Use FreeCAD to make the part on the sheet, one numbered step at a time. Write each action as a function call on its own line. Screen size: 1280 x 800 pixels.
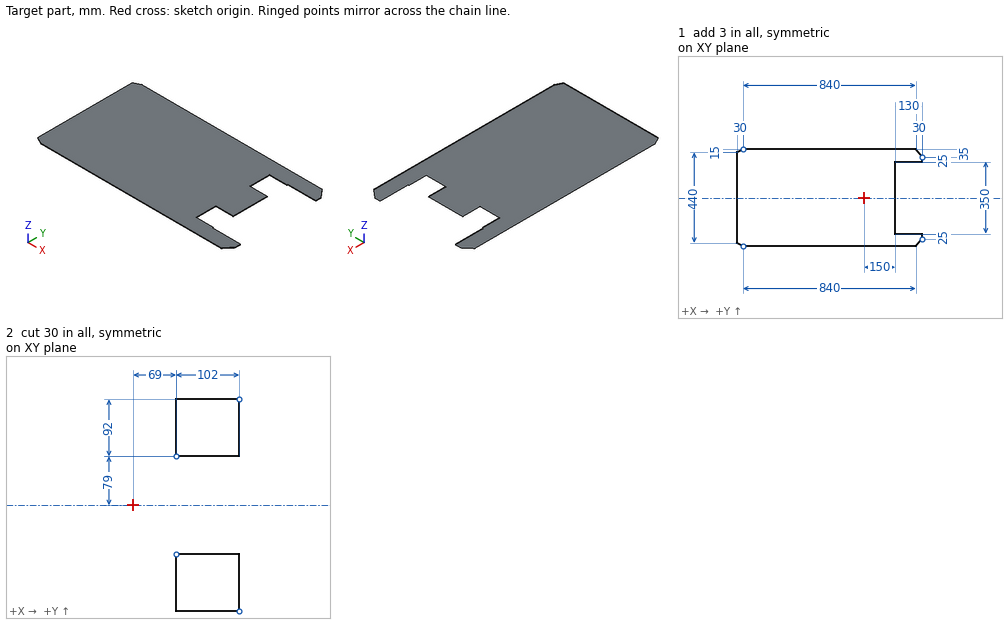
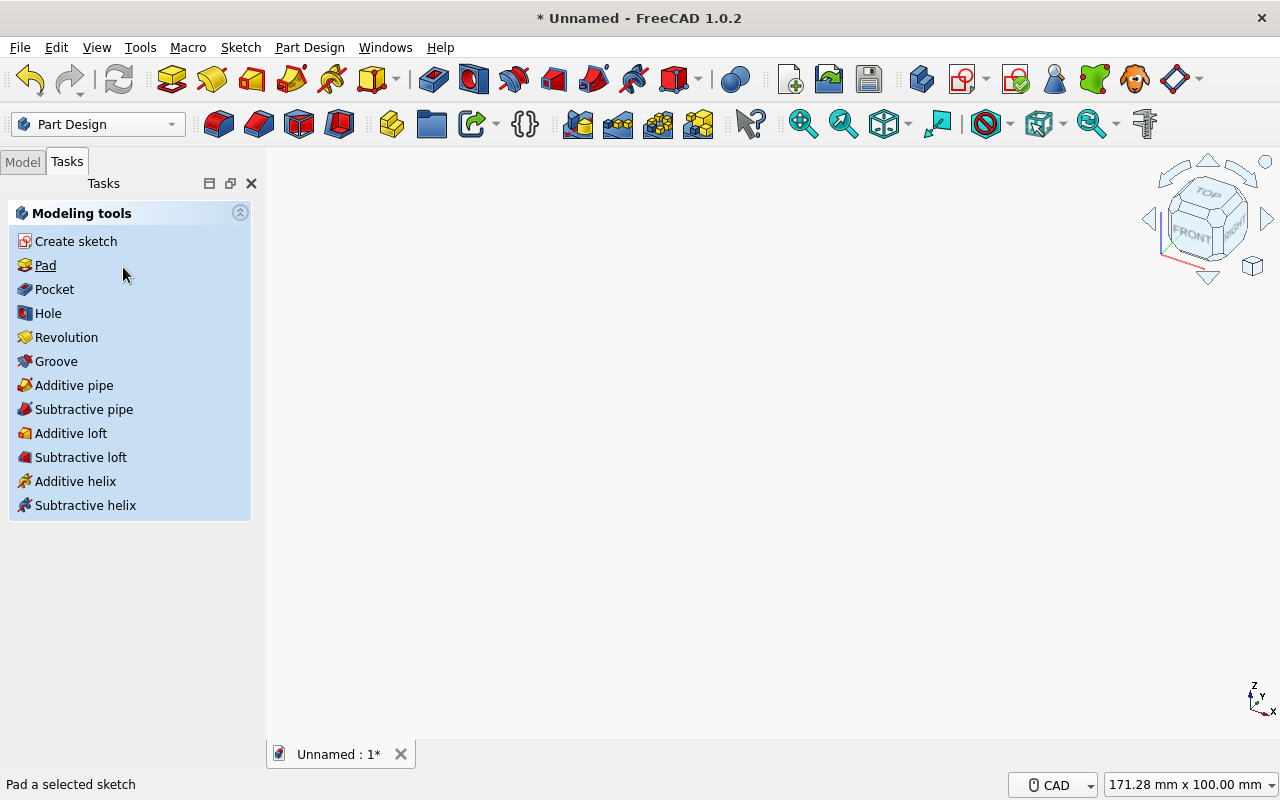
click(172, 80)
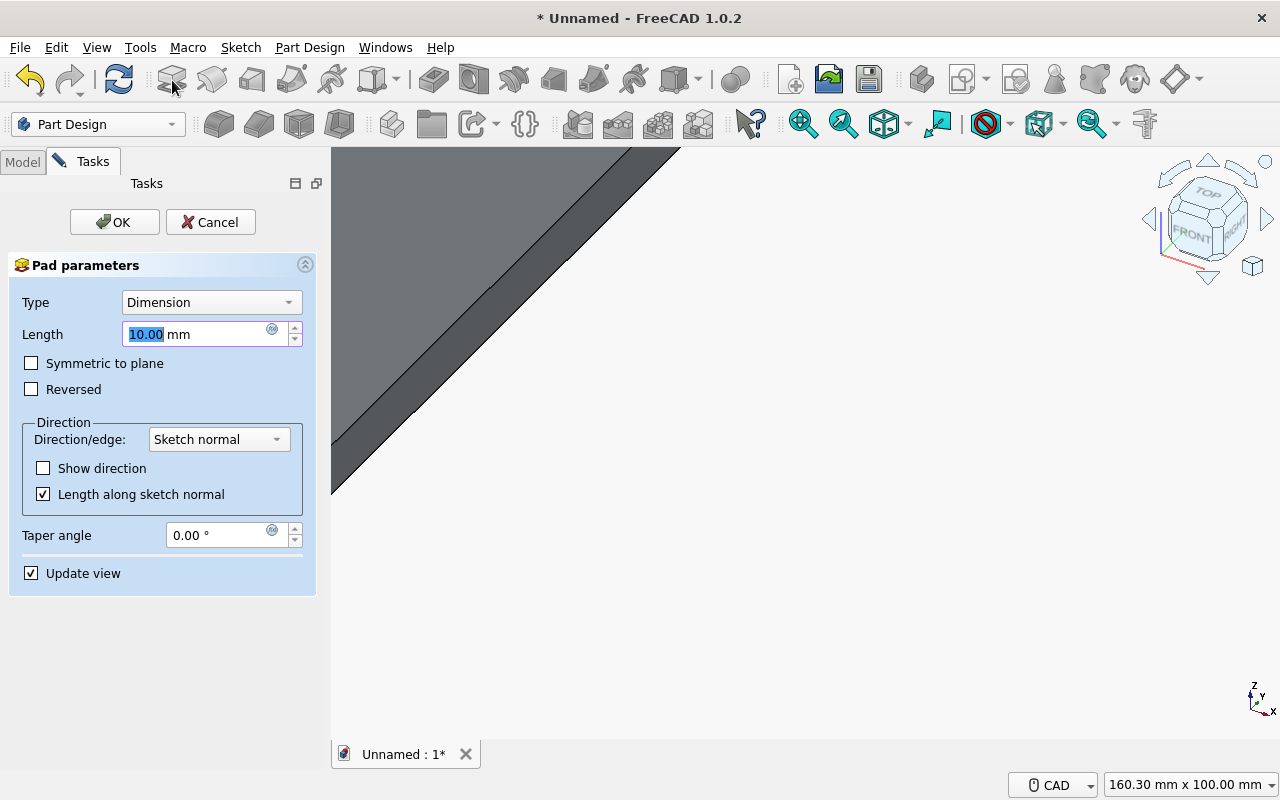
text(3)
key(Tab)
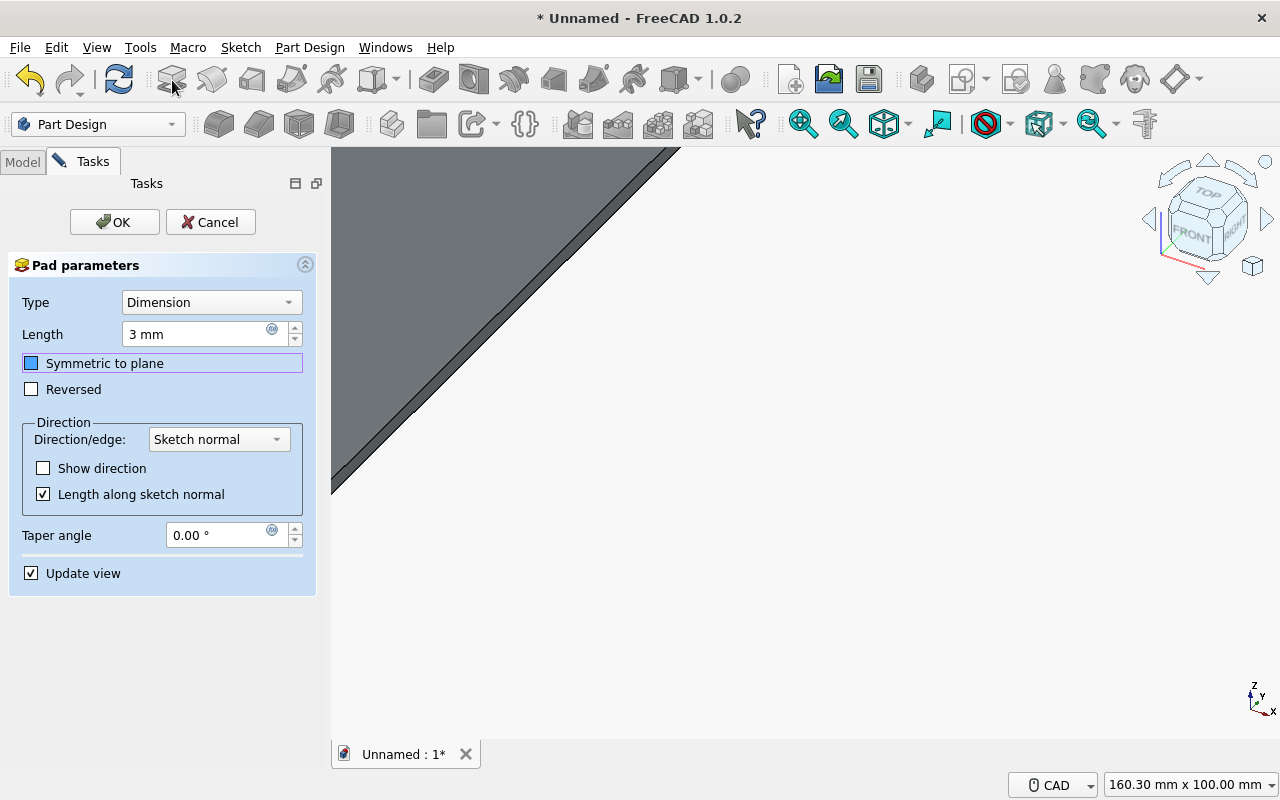
click(30, 363)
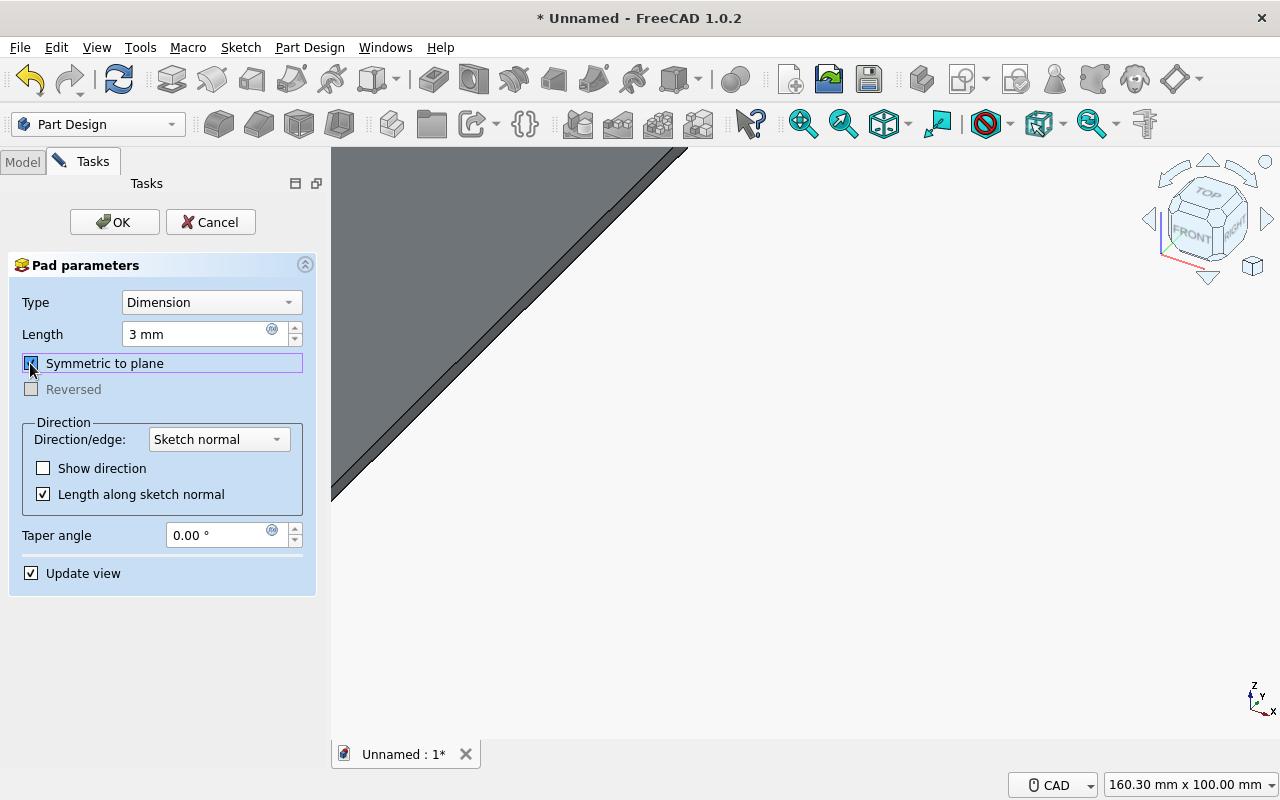
click(115, 222)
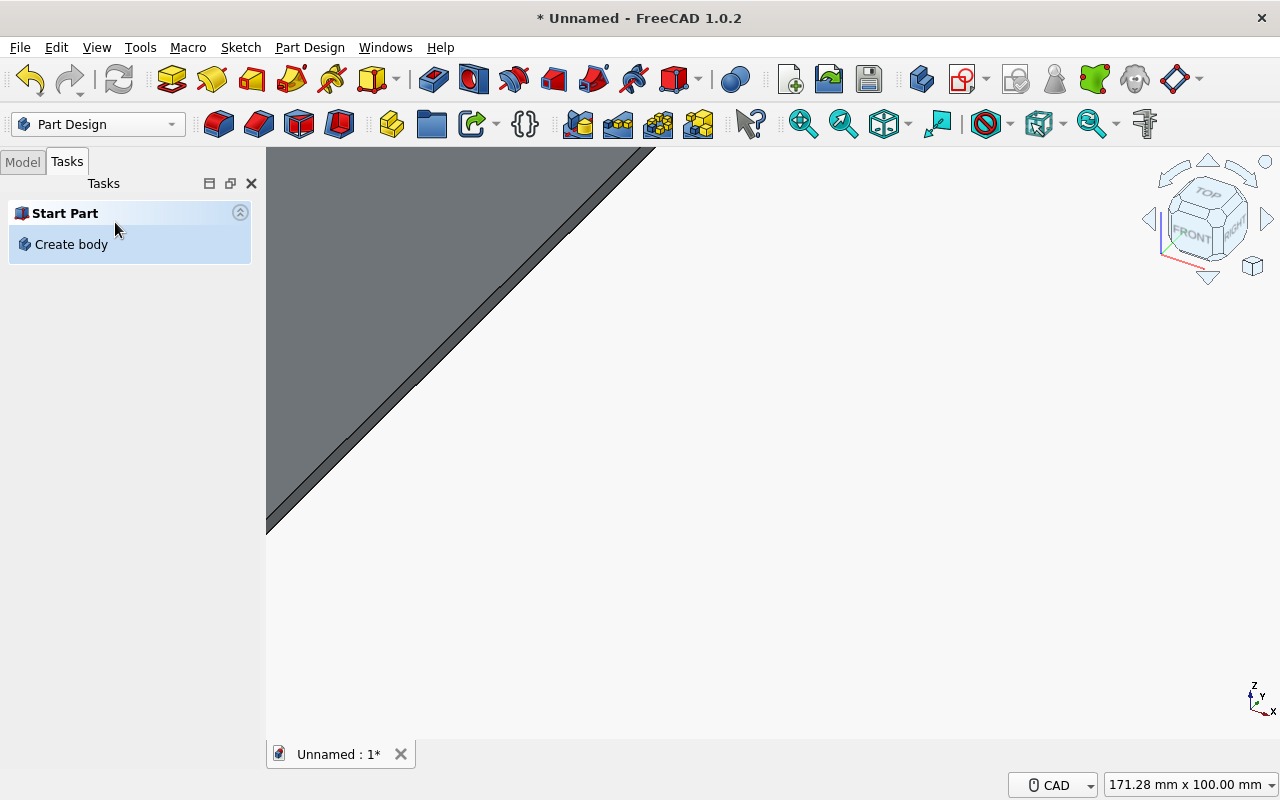
click(804, 124)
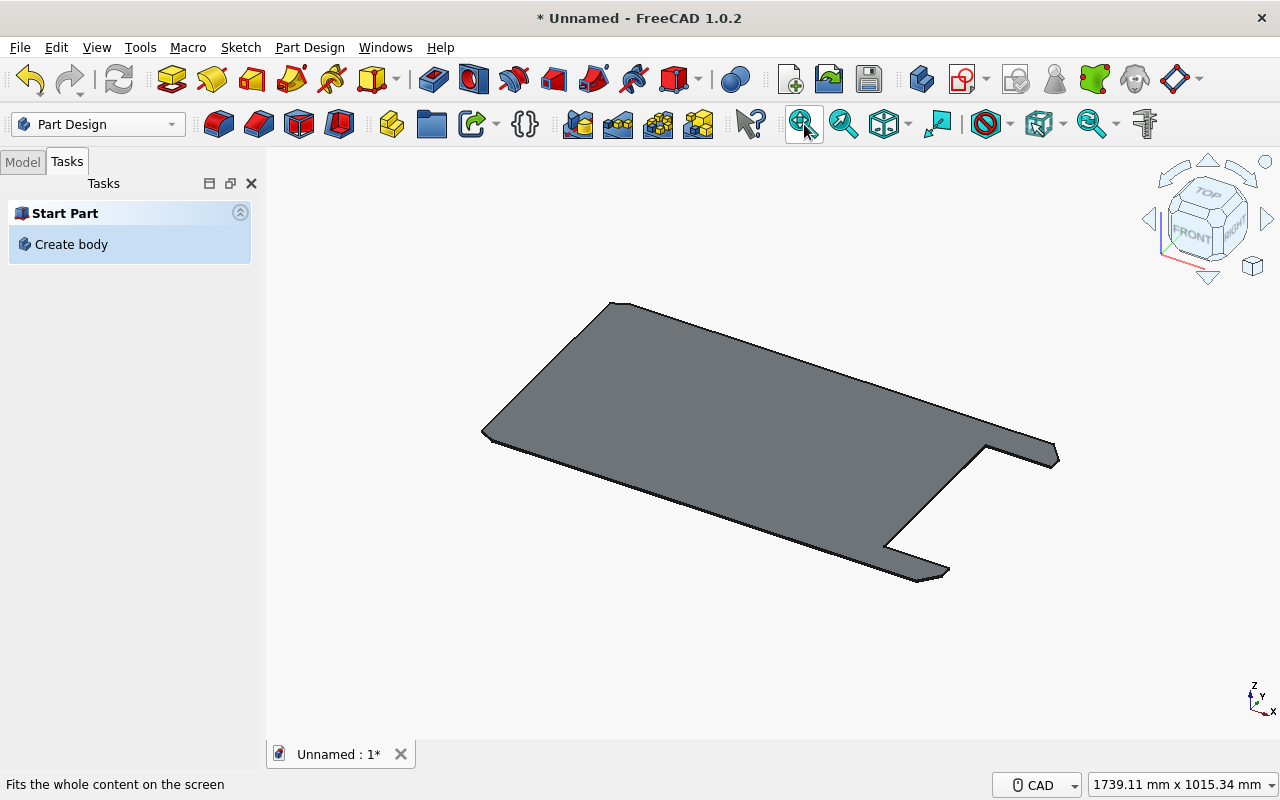
click(962, 80)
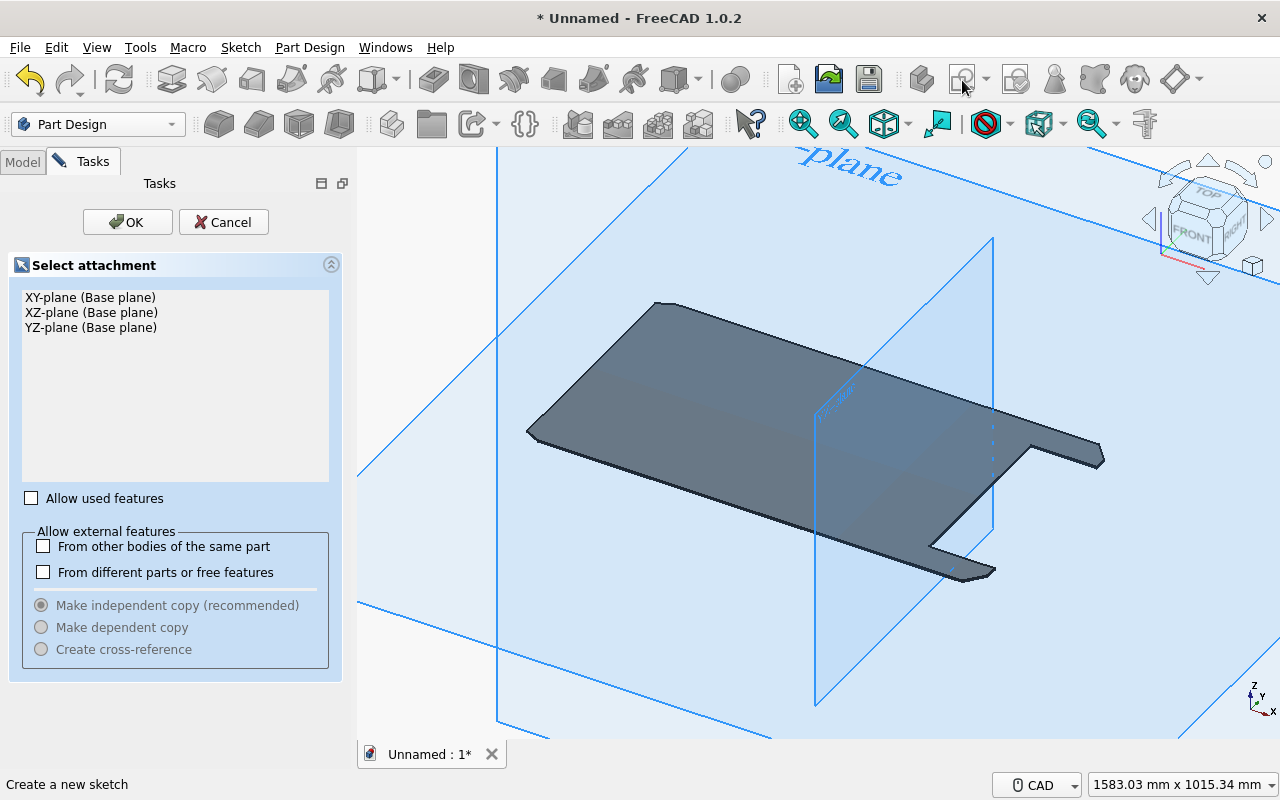
click(82, 298)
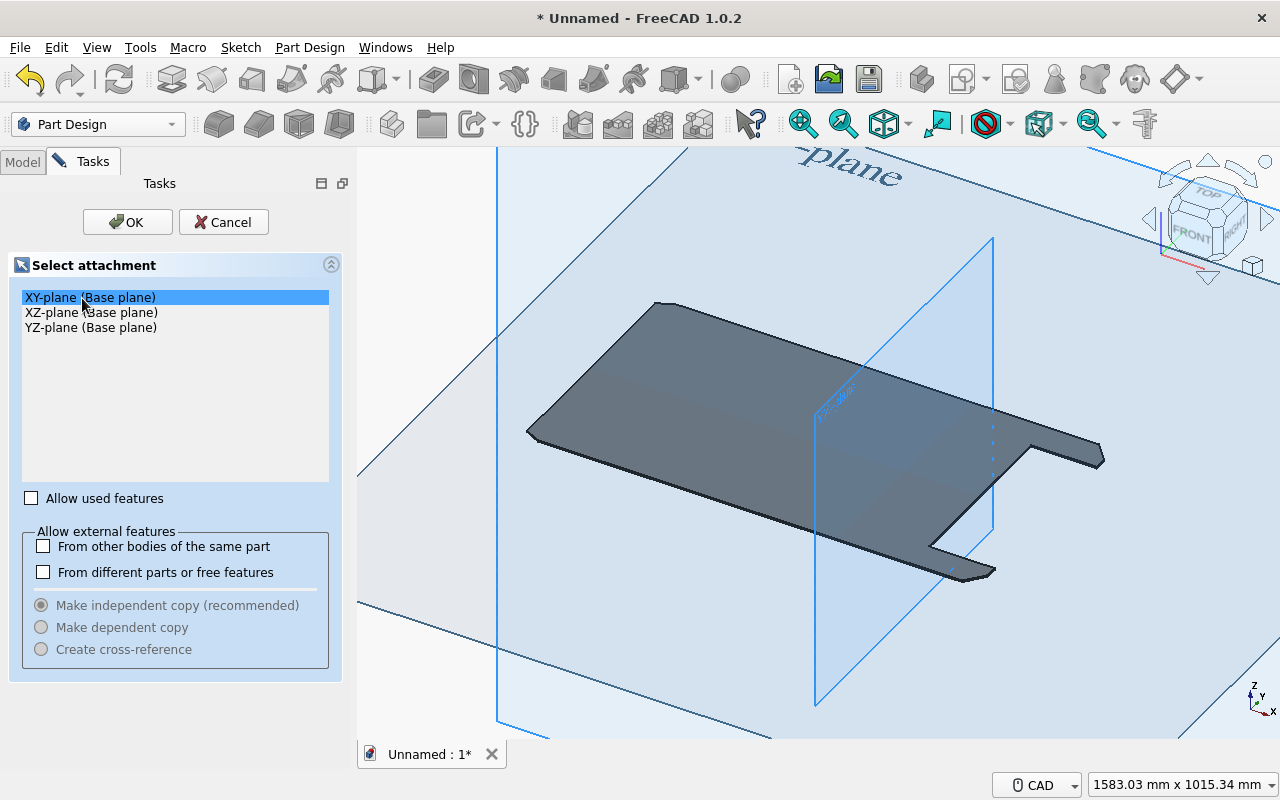
click(128, 222)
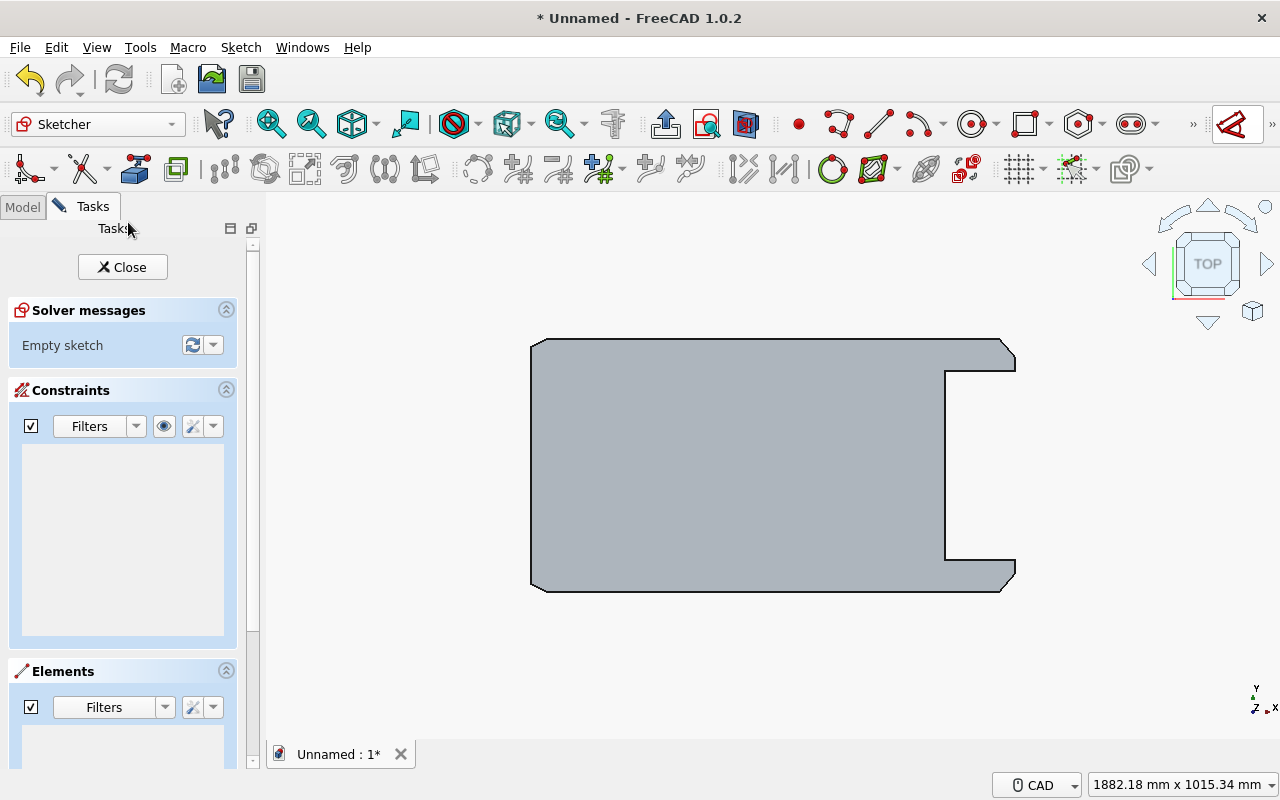
click(746, 124)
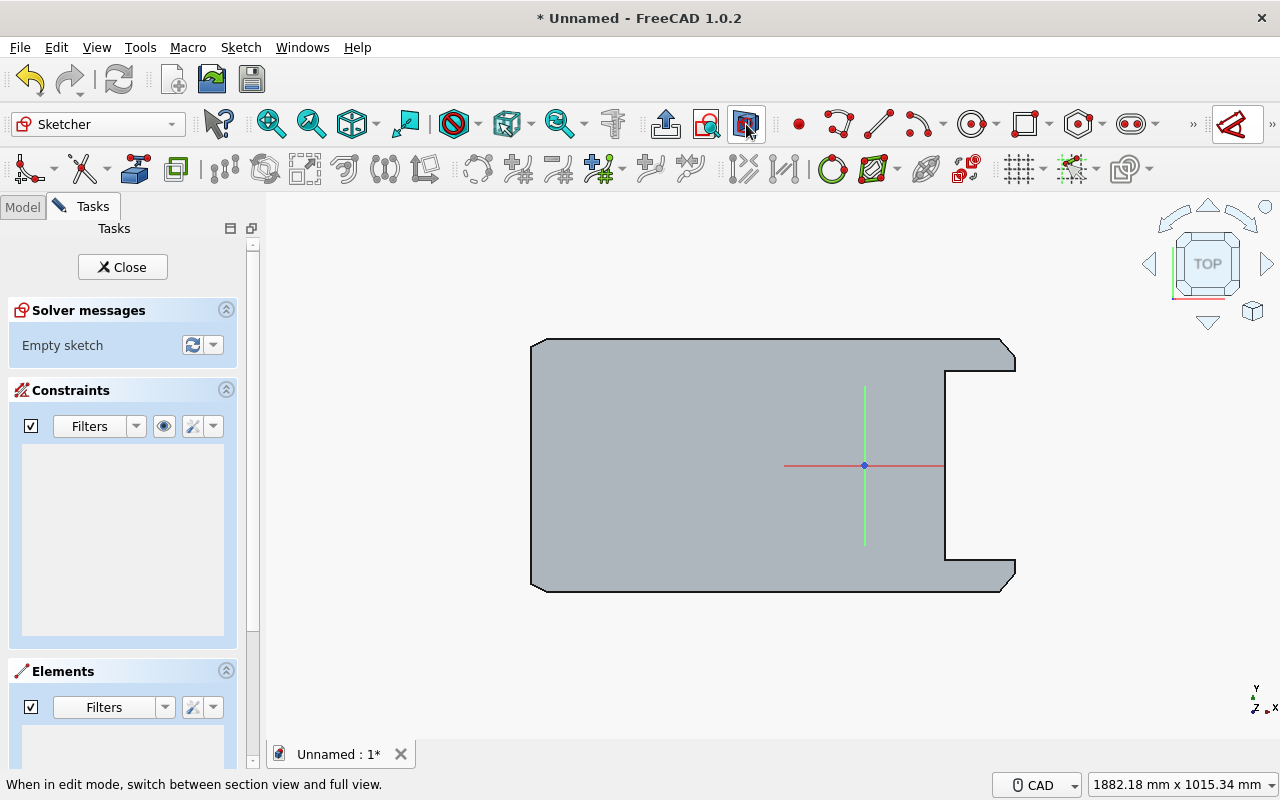
scroll(1115, 466, up, 3)